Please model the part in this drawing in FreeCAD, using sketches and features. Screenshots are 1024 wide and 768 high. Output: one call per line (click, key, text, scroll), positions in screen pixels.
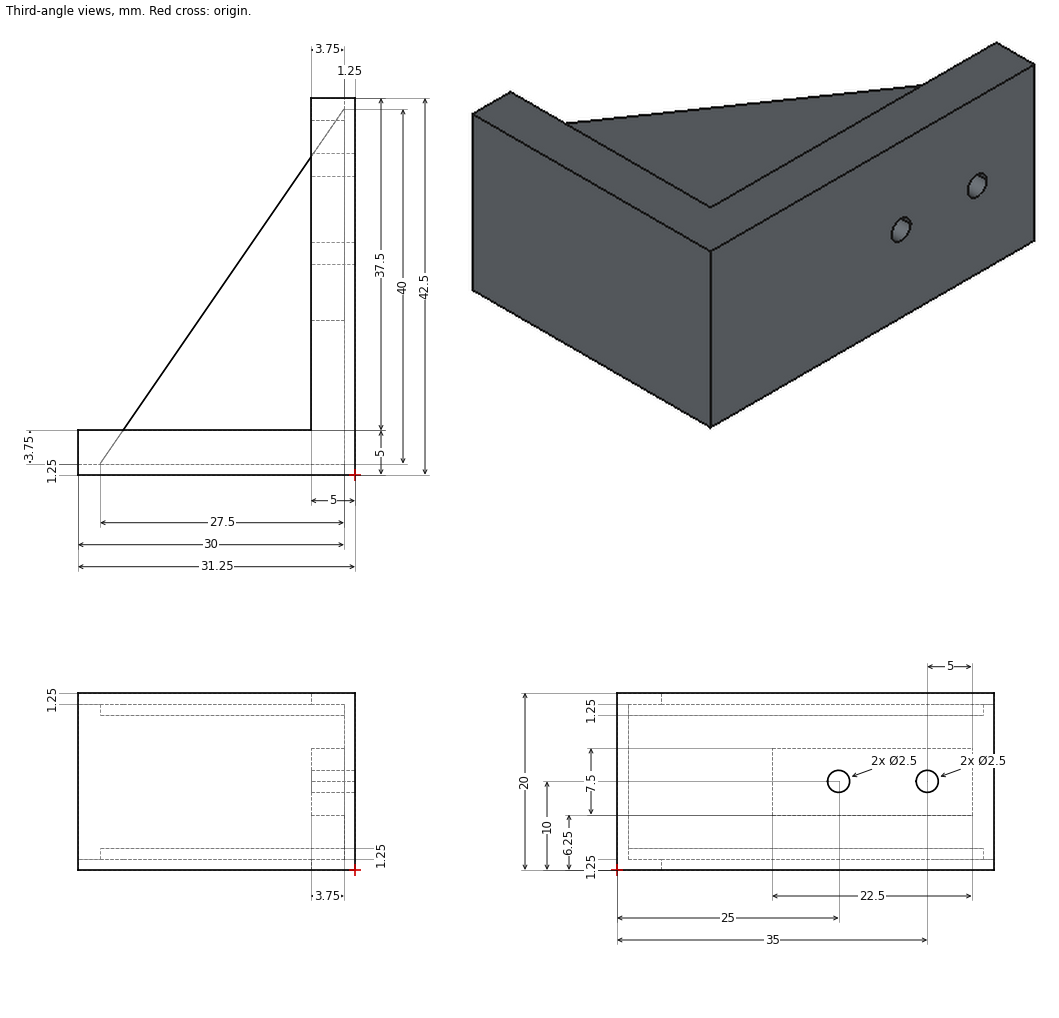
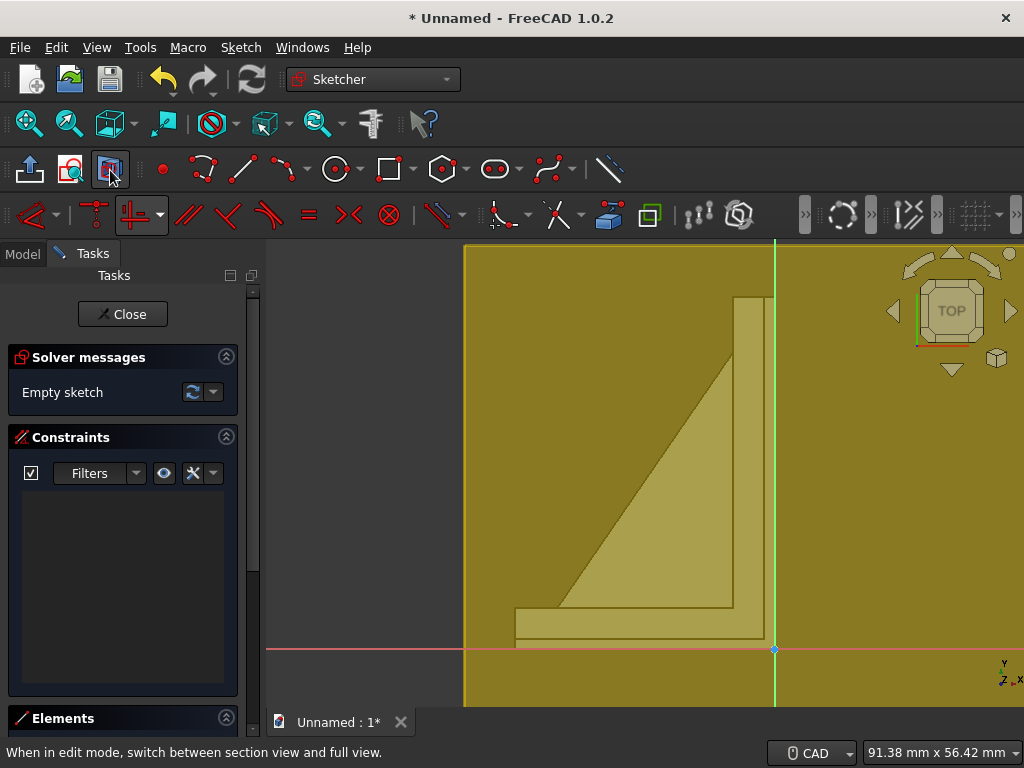
click(204, 170)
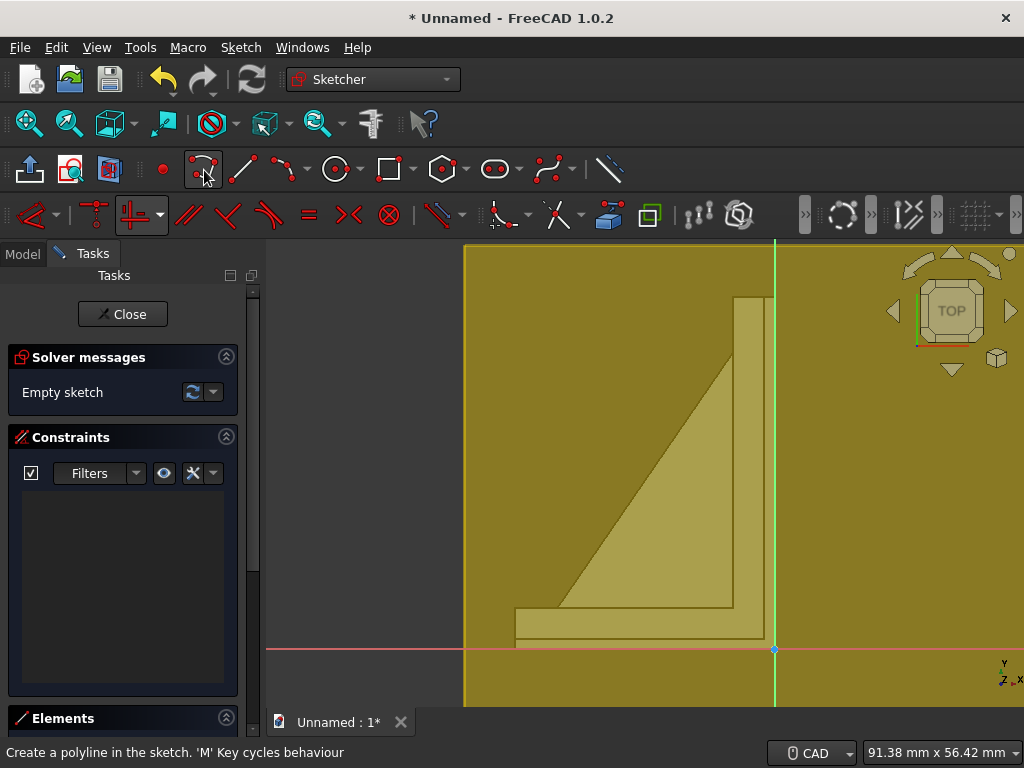
scroll(764, 639, up, 3)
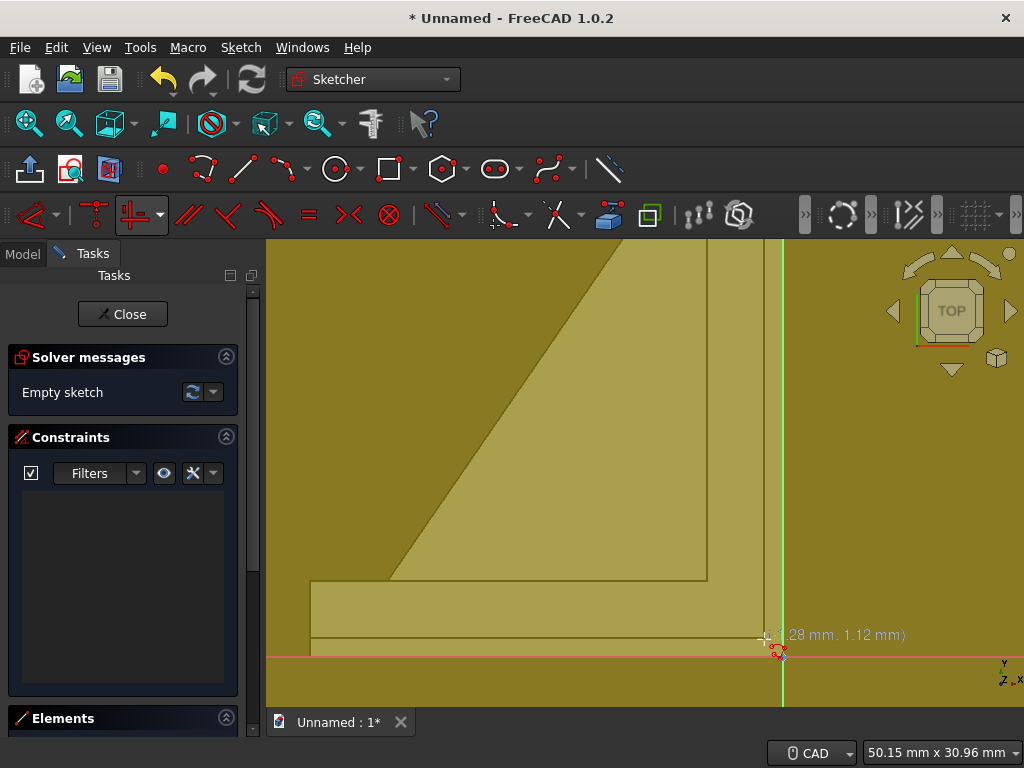
click(764, 638)
click(348, 638)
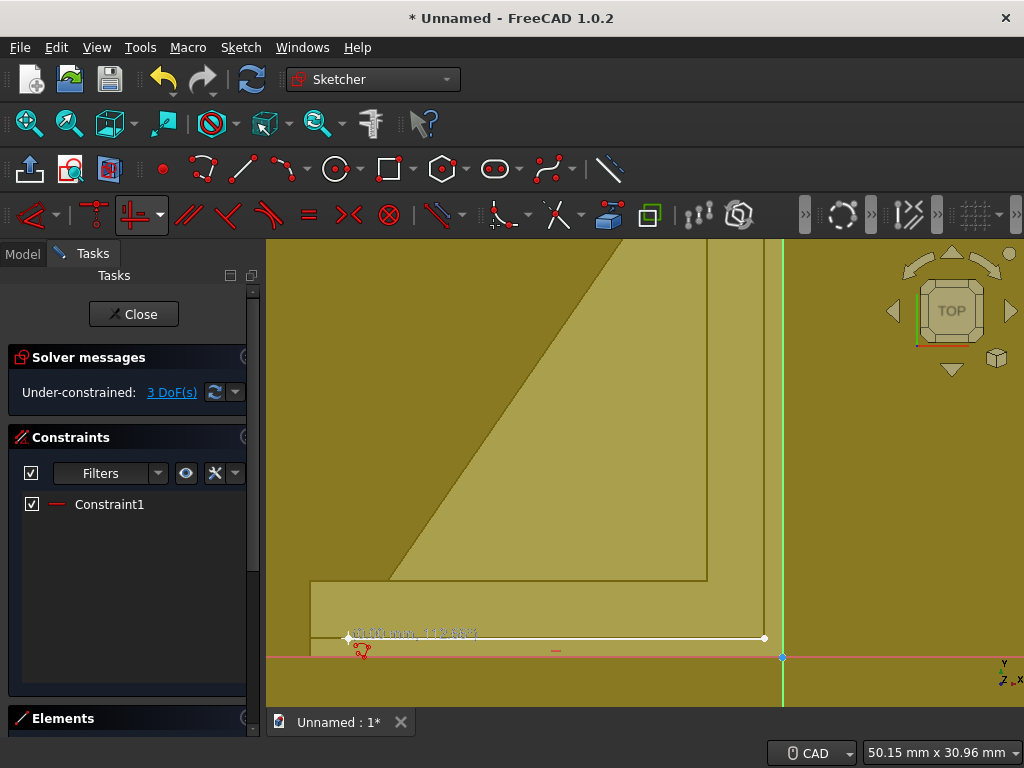
scroll(585, 577, down, 4)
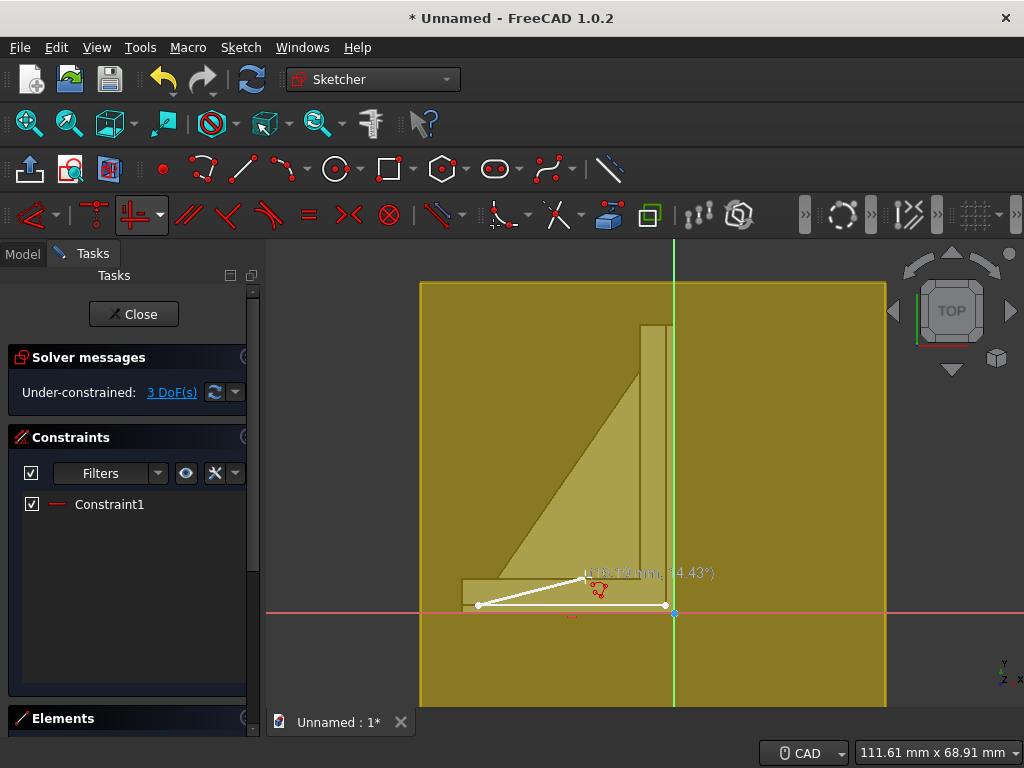
scroll(666, 333, up, 4)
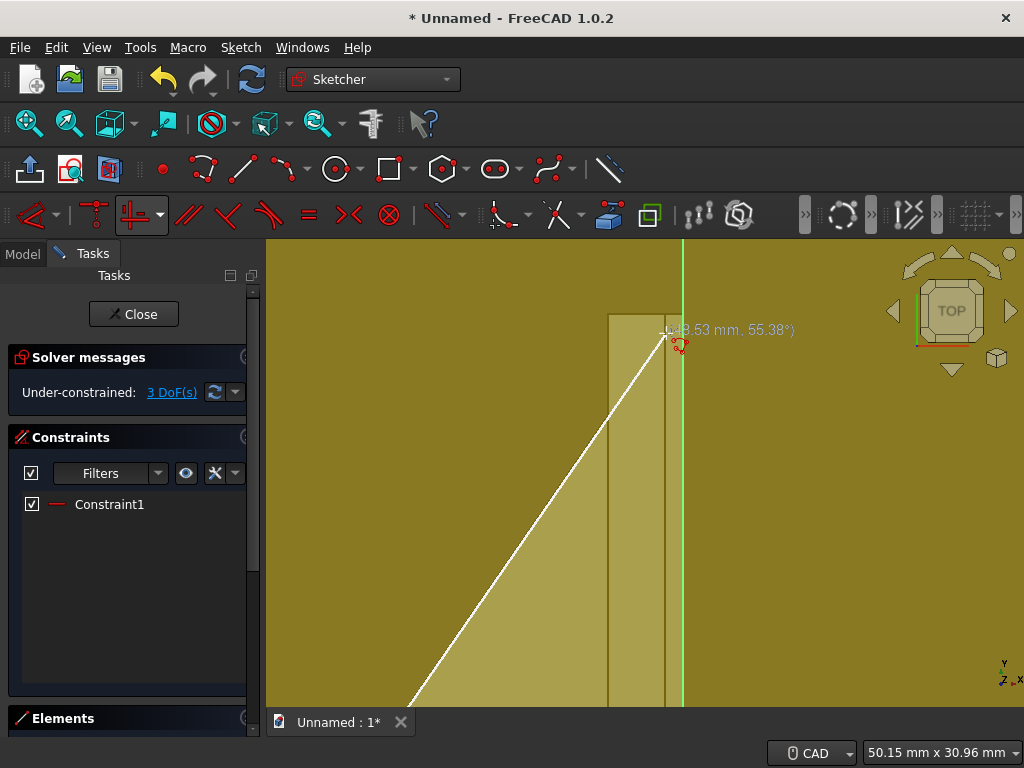
click(665, 333)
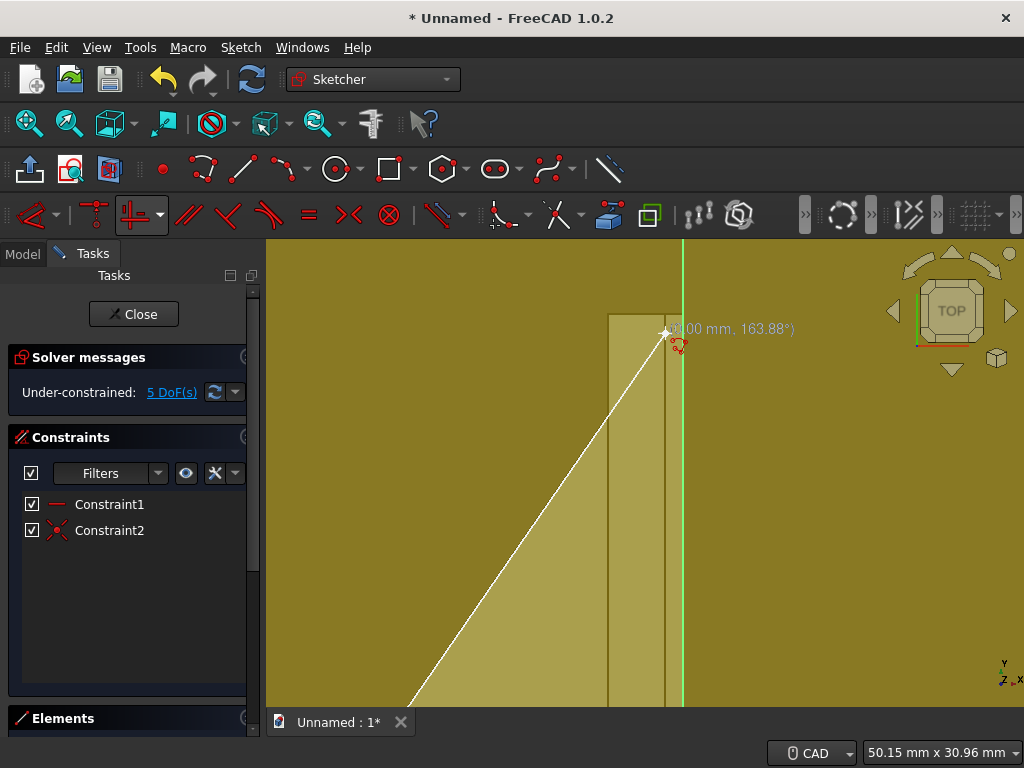
scroll(667, 333, down, 4)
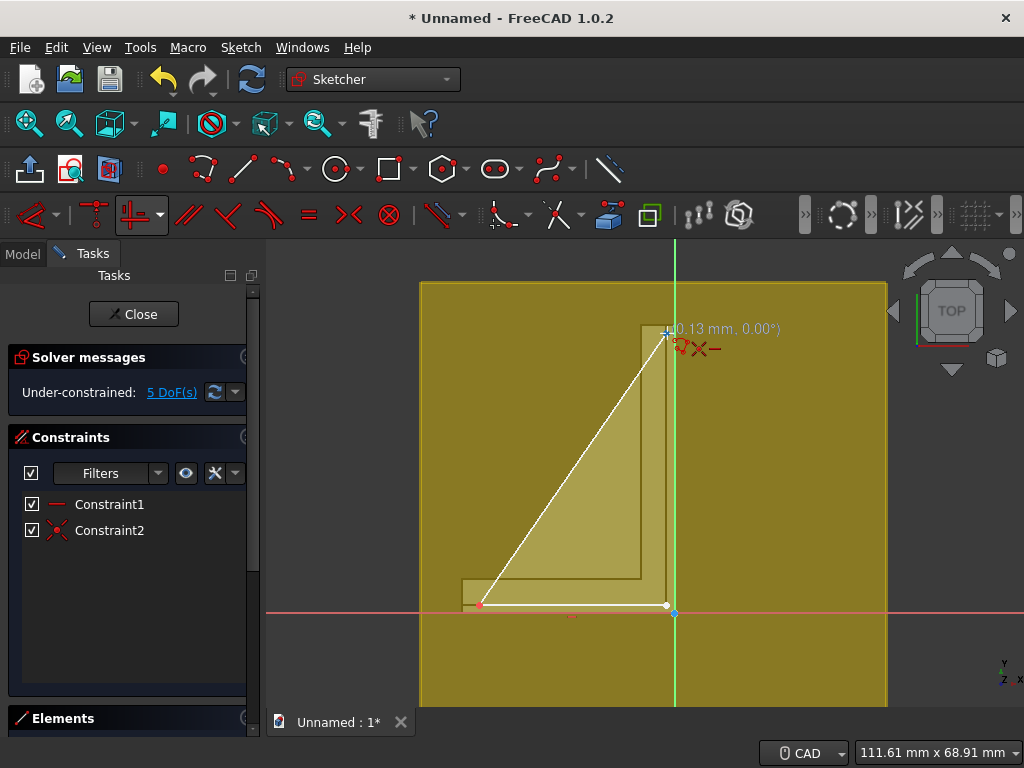
scroll(666, 605, up, 4)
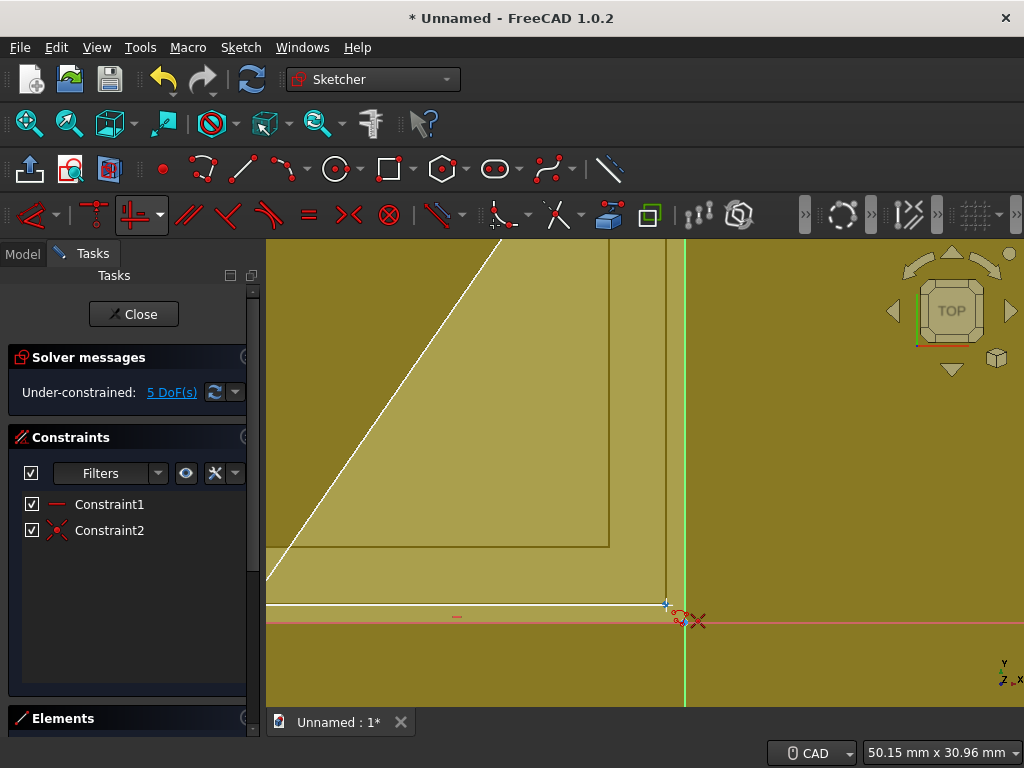
click(666, 605)
key(Escape)
key(Escape)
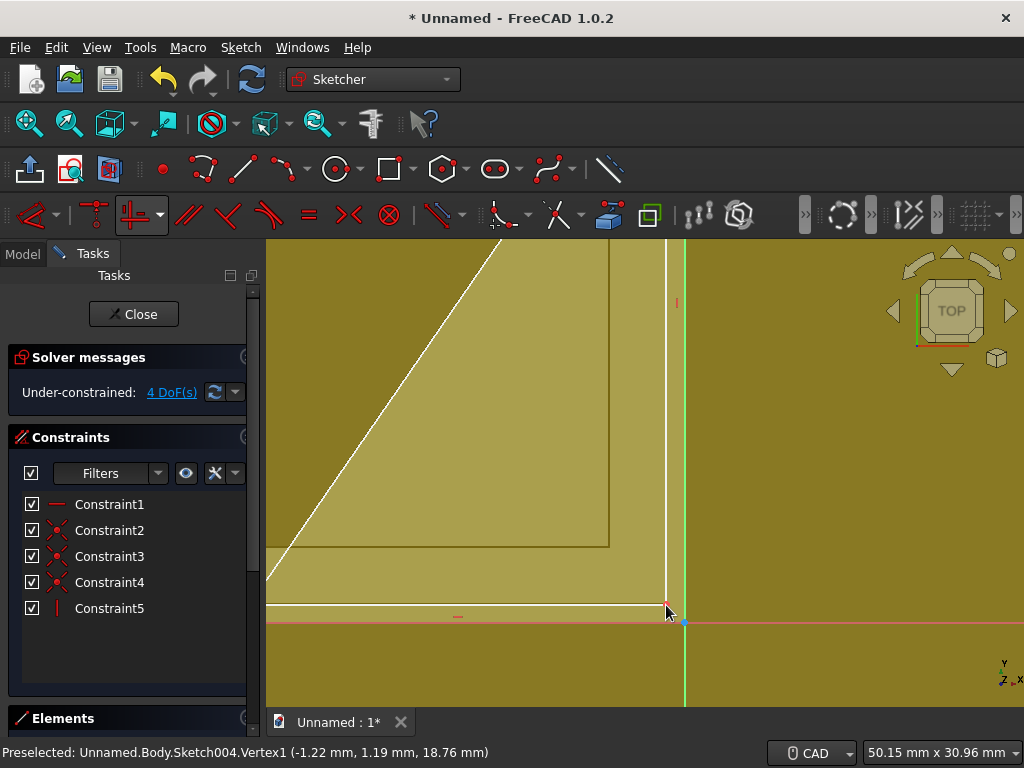
click(32, 216)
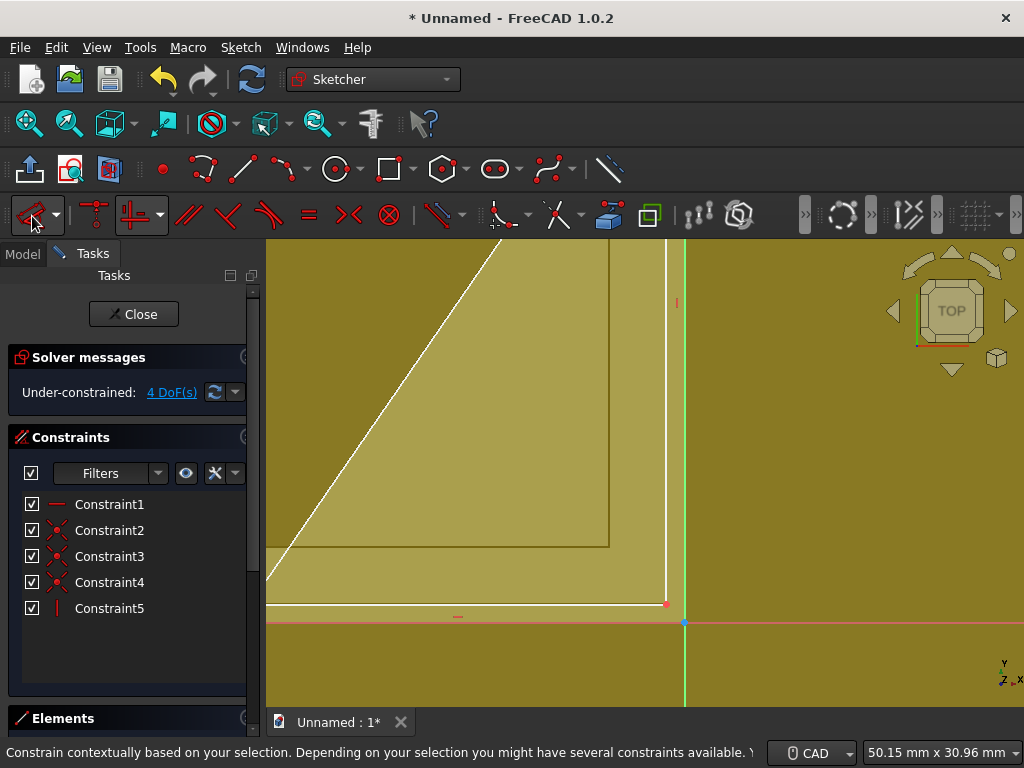
click(666, 423)
click(700, 436)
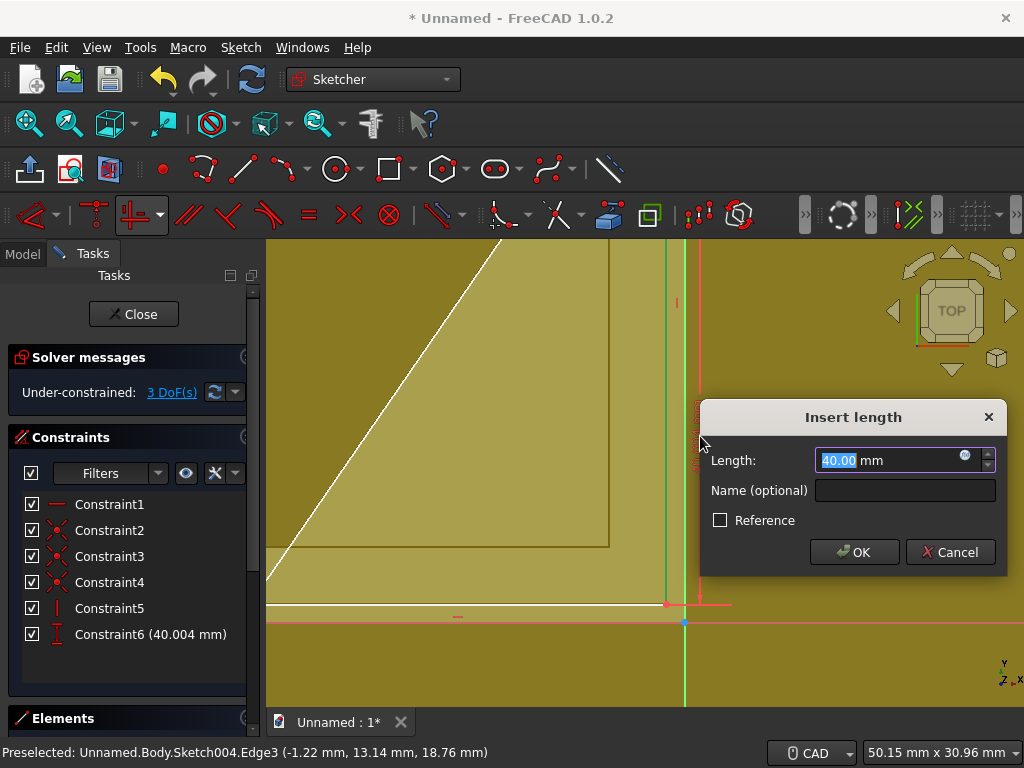
text(40)
key(Return)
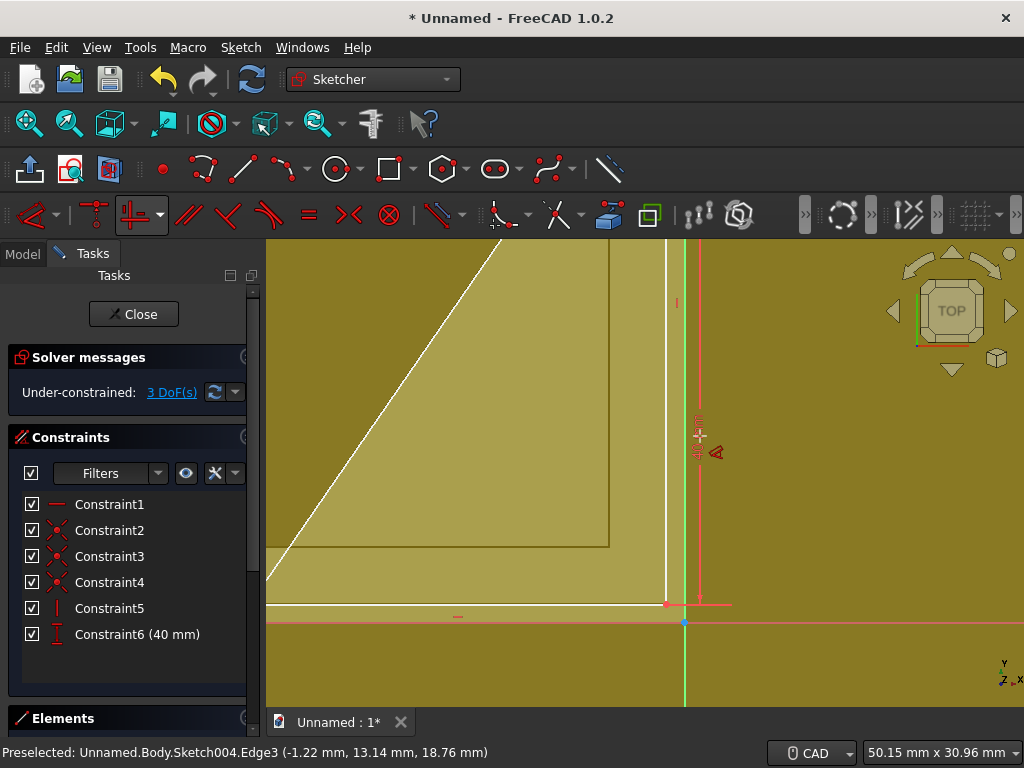
click(541, 605)
click(480, 639)